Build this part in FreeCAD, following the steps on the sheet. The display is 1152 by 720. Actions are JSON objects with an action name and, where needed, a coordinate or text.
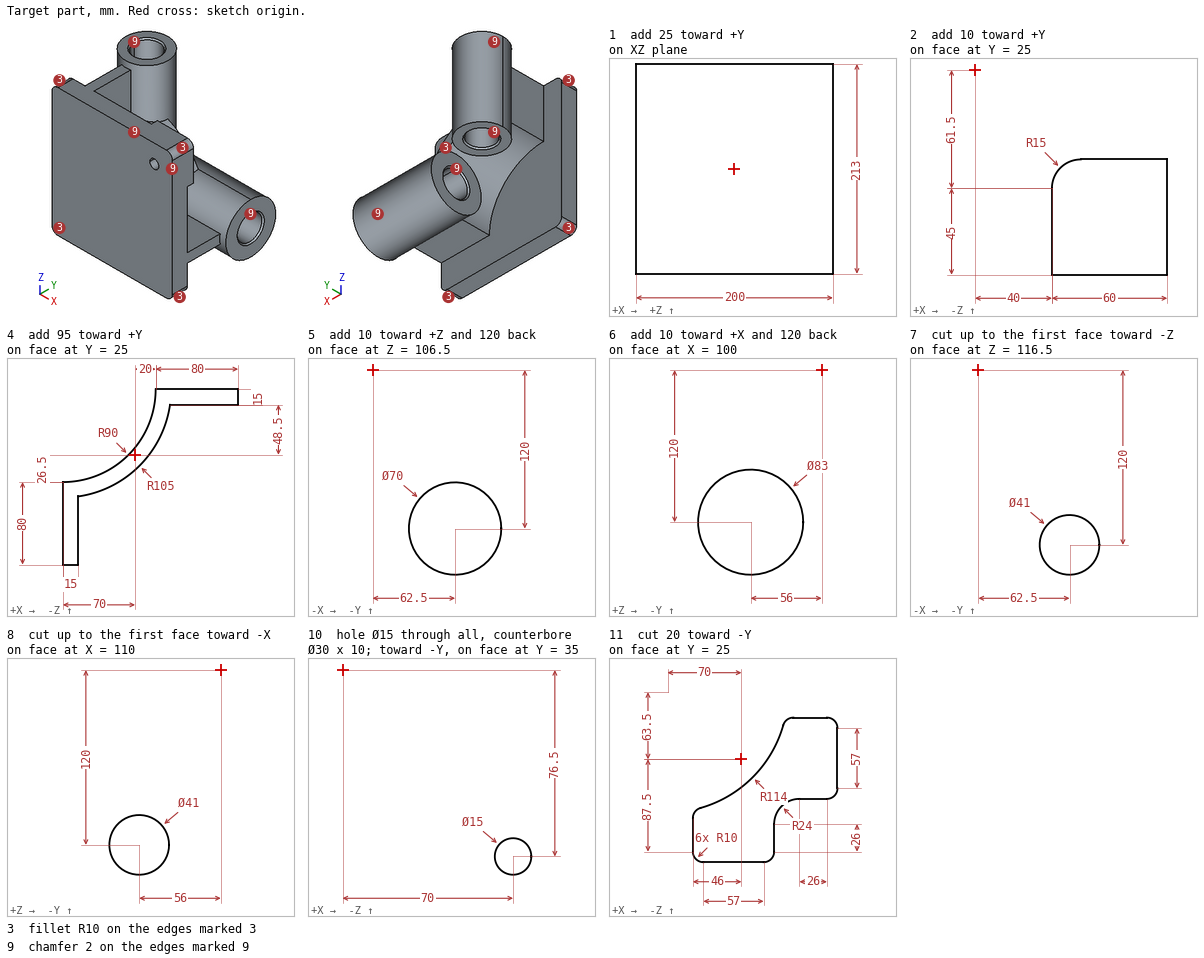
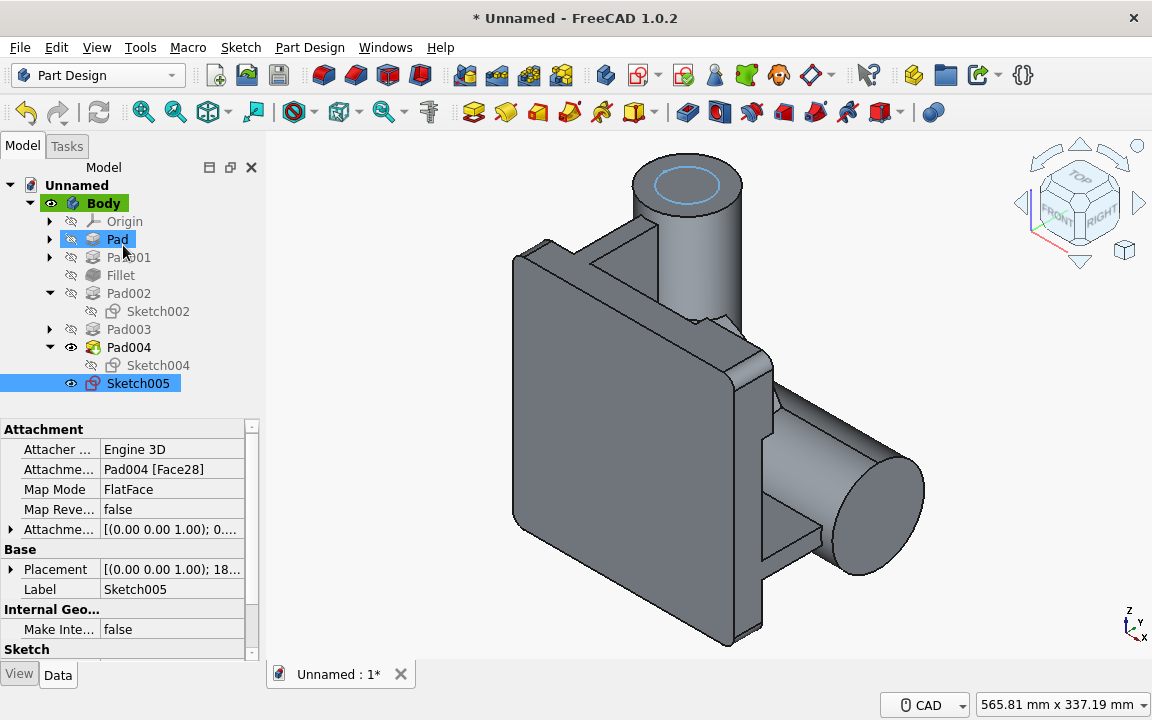
{"action": "left_click", "coordinate": [688, 112]}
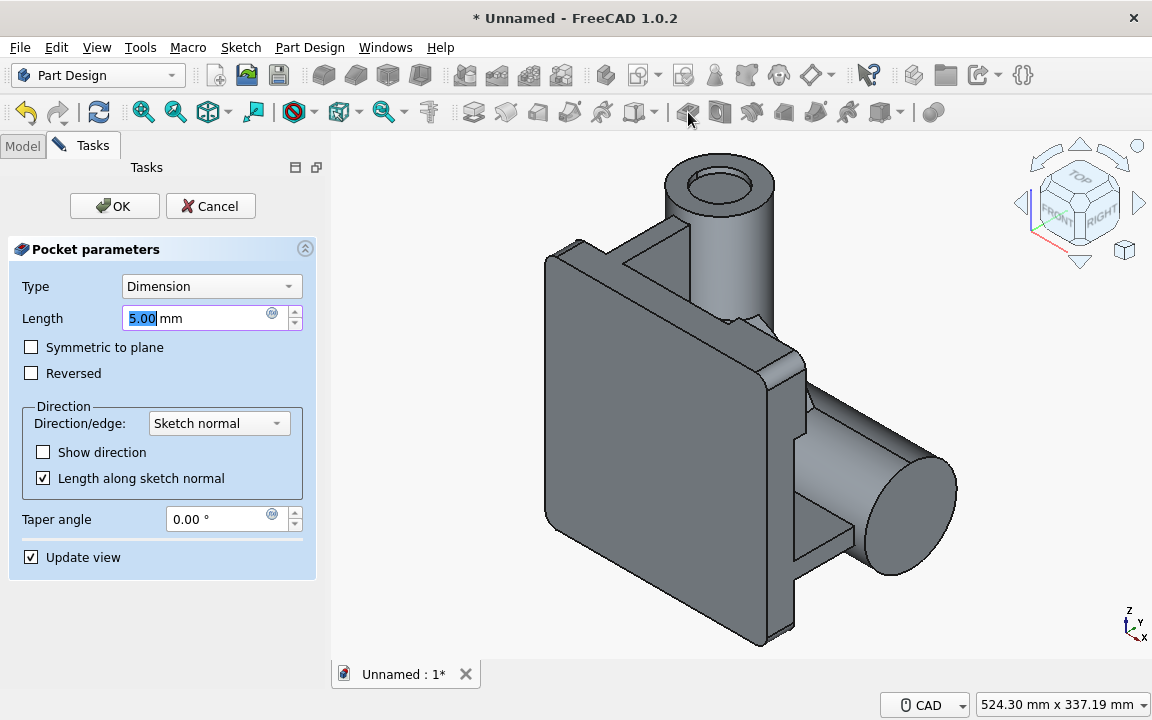
{"action": "left_click", "coordinate": [212, 286]}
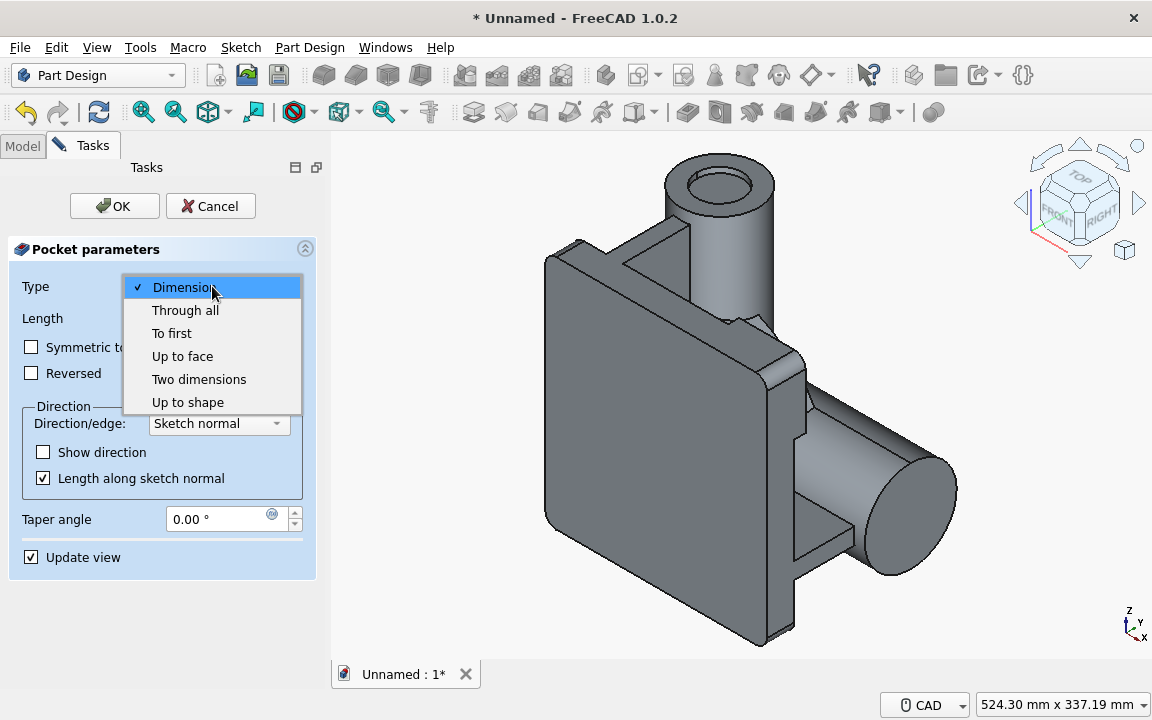
{"action": "left_click", "coordinate": [212, 334]}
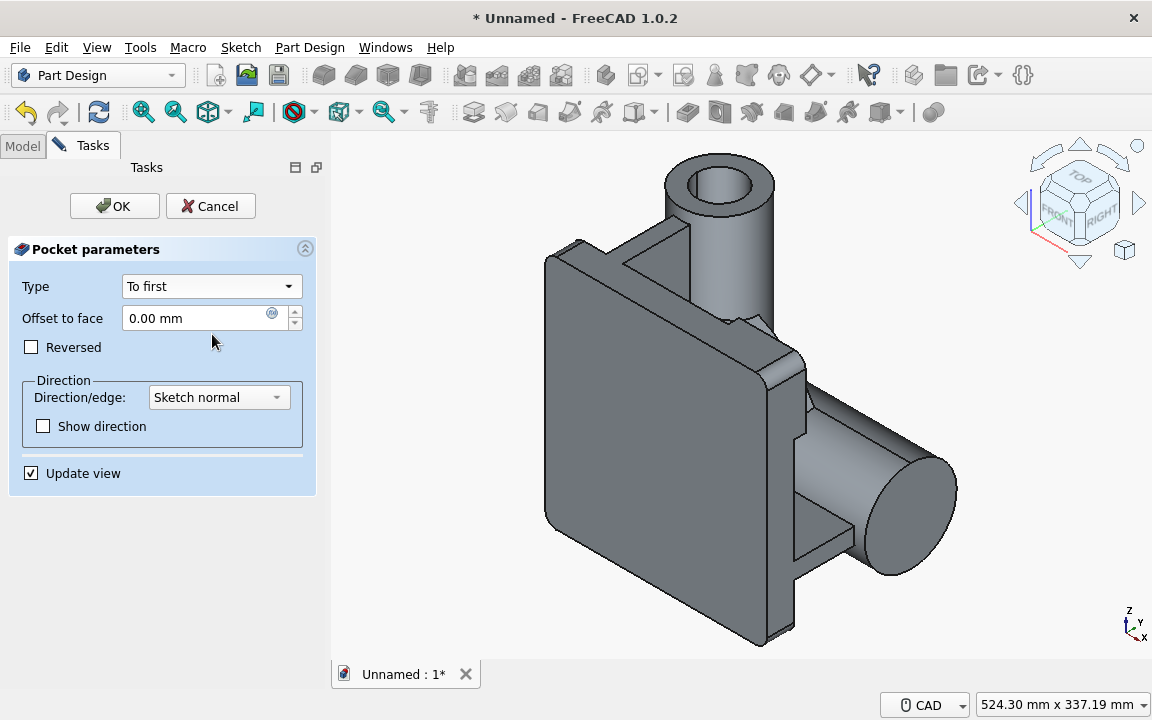
{"action": "left_click", "coordinate": [115, 206]}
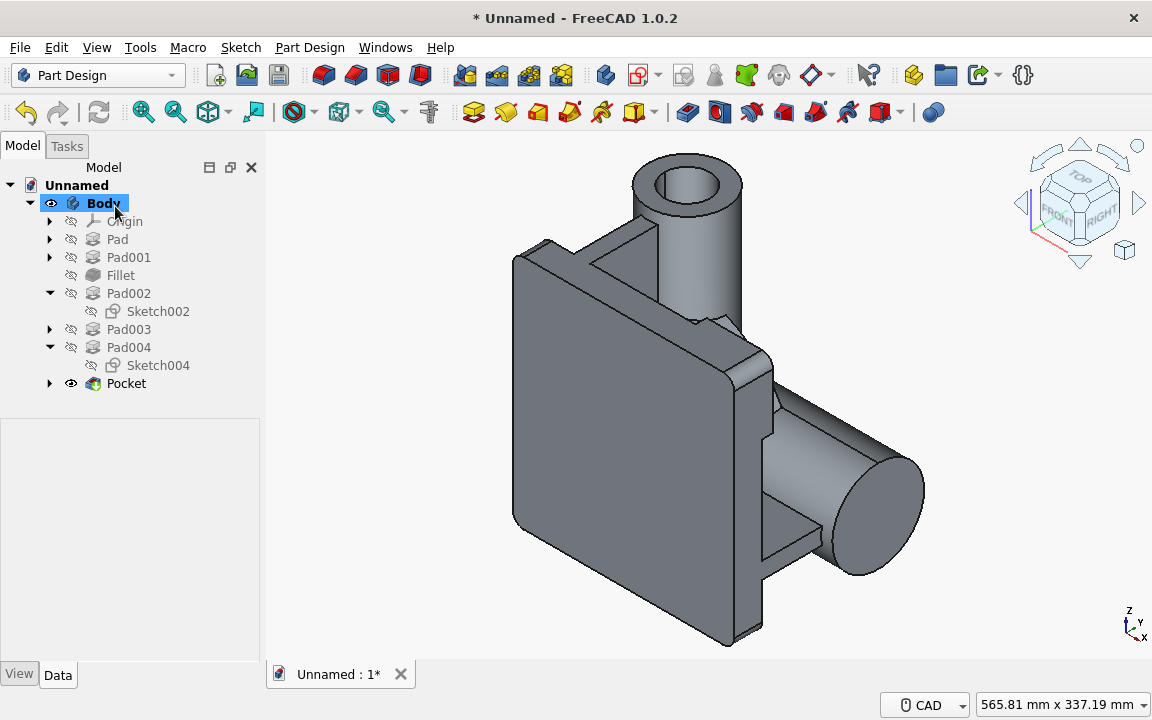
{"action": "left_click", "coordinate": [878, 515]}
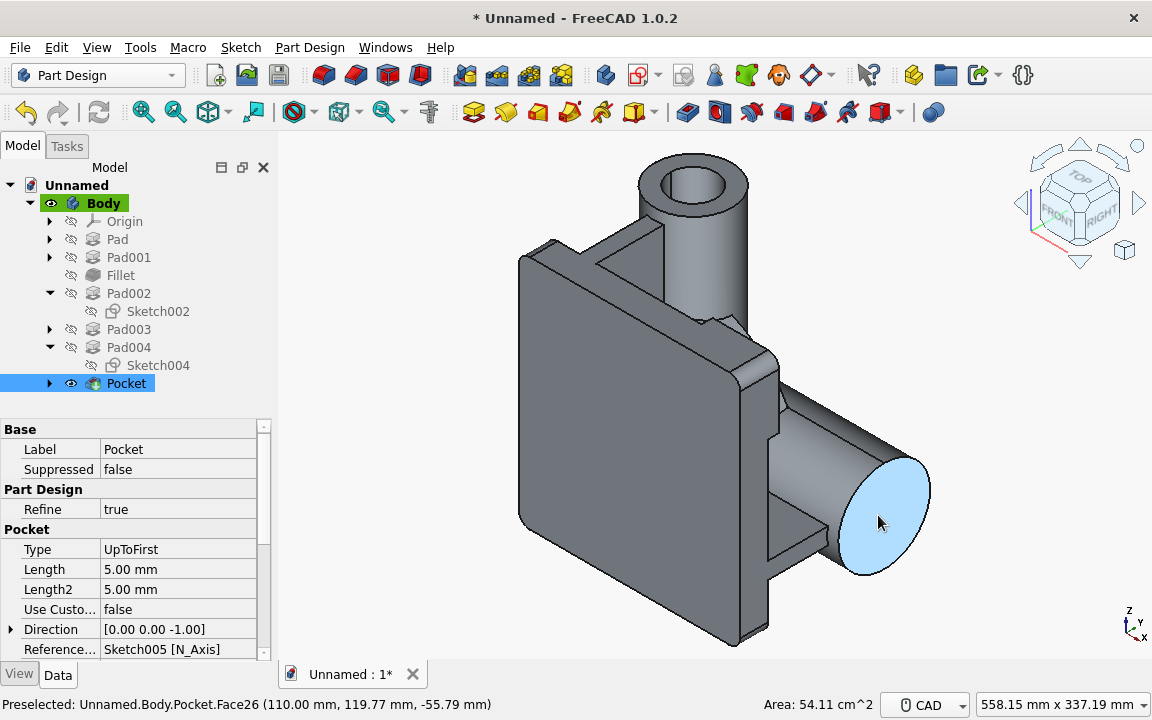
{"action": "left_click", "coordinate": [638, 76]}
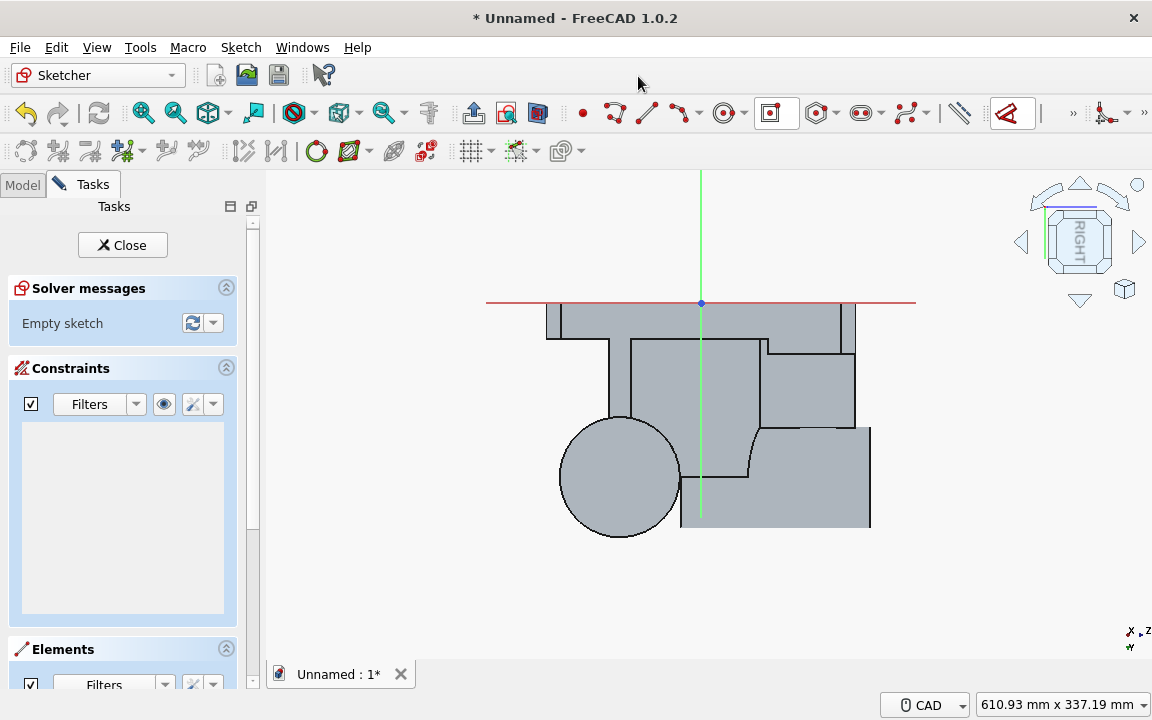
{"action": "scroll", "coordinate": [615, 493], "scroll_direction": "up", "scroll_amount": 8}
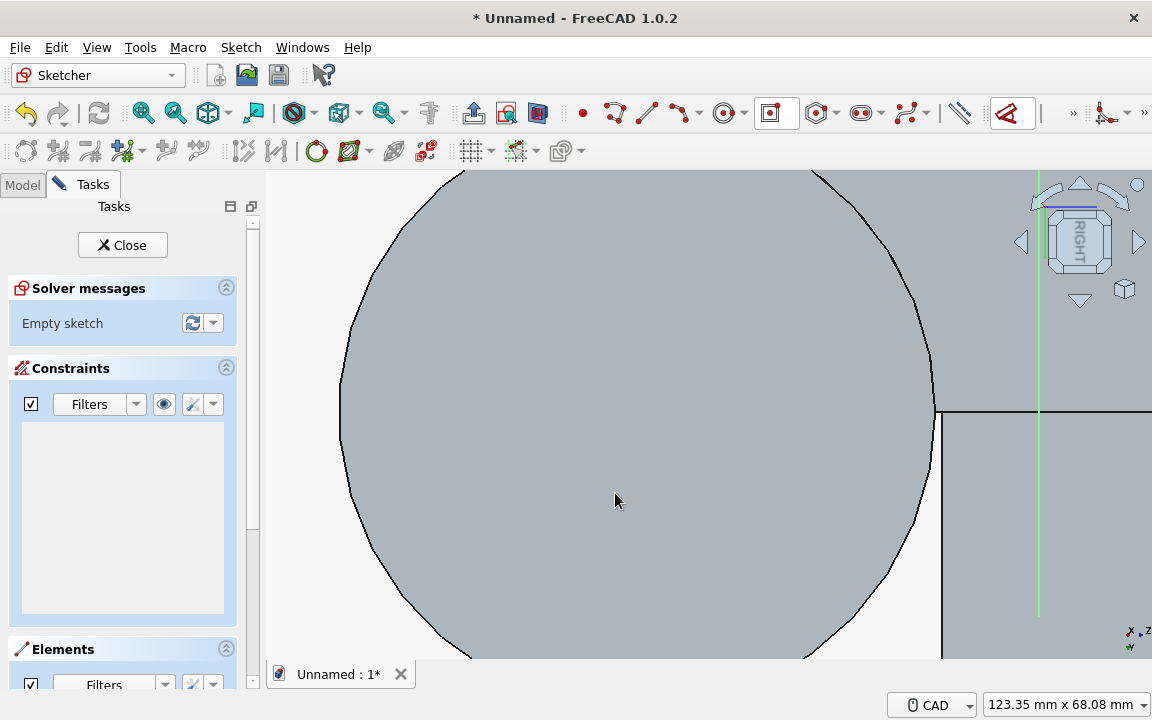
{"action": "left_click", "coordinate": [724, 114]}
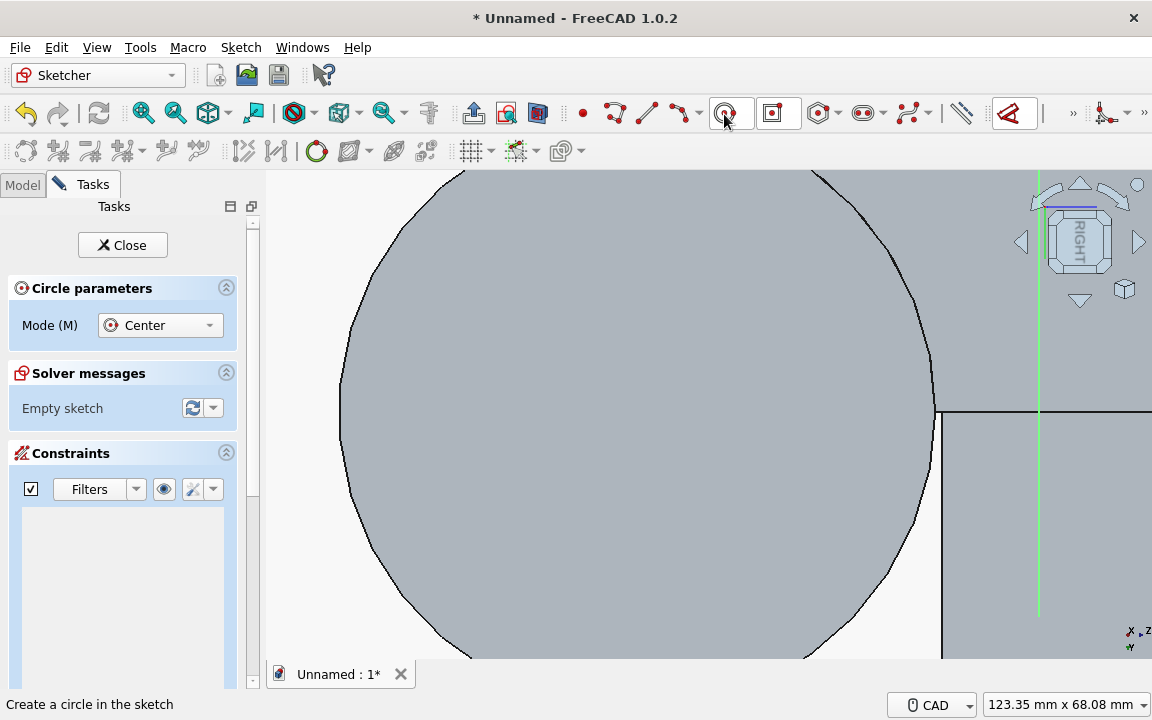
{"action": "left_click", "coordinate": [637, 412]}
{"action": "mouse_move", "coordinate": [741, 308]}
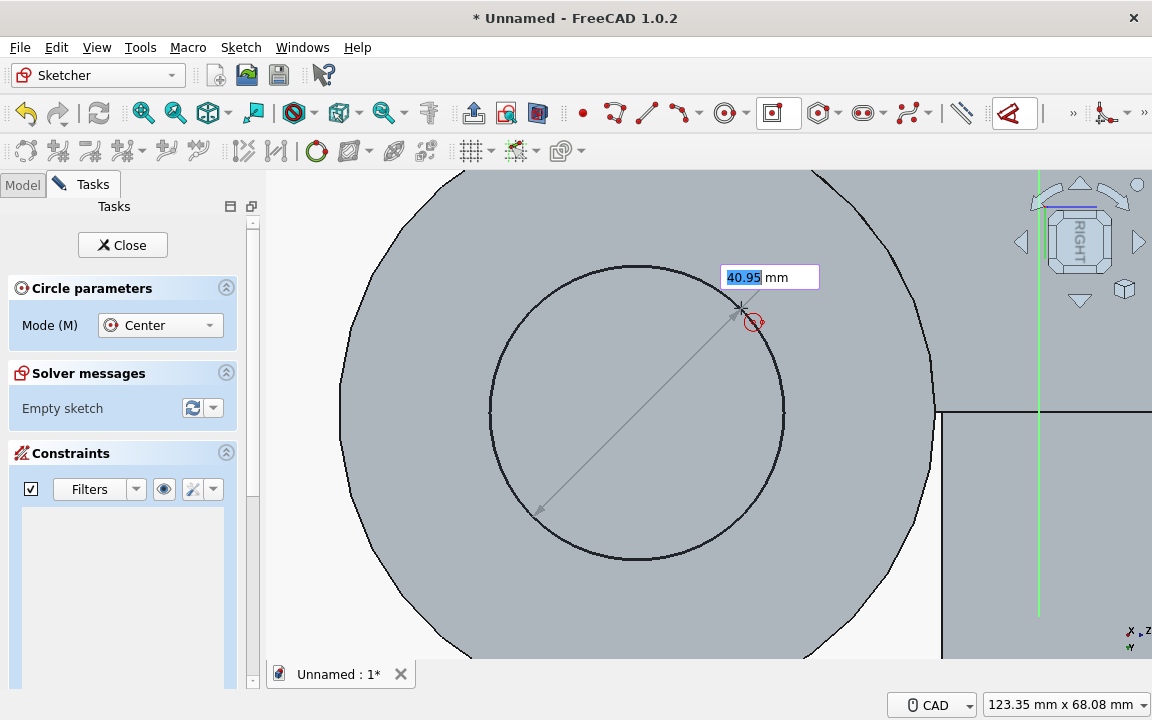
{"action": "type", "text": "41"}
{"action": "key", "text": "Return"}
{"action": "key", "text": "Escape"}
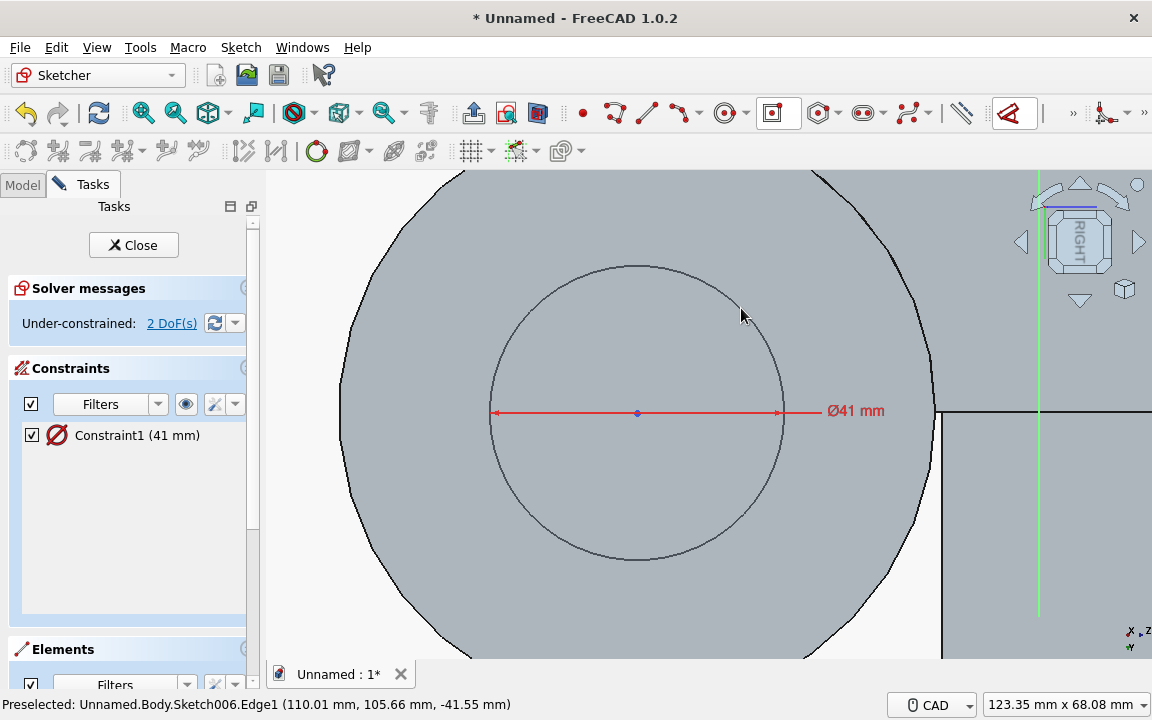
{"action": "left_click", "coordinate": [637, 413]}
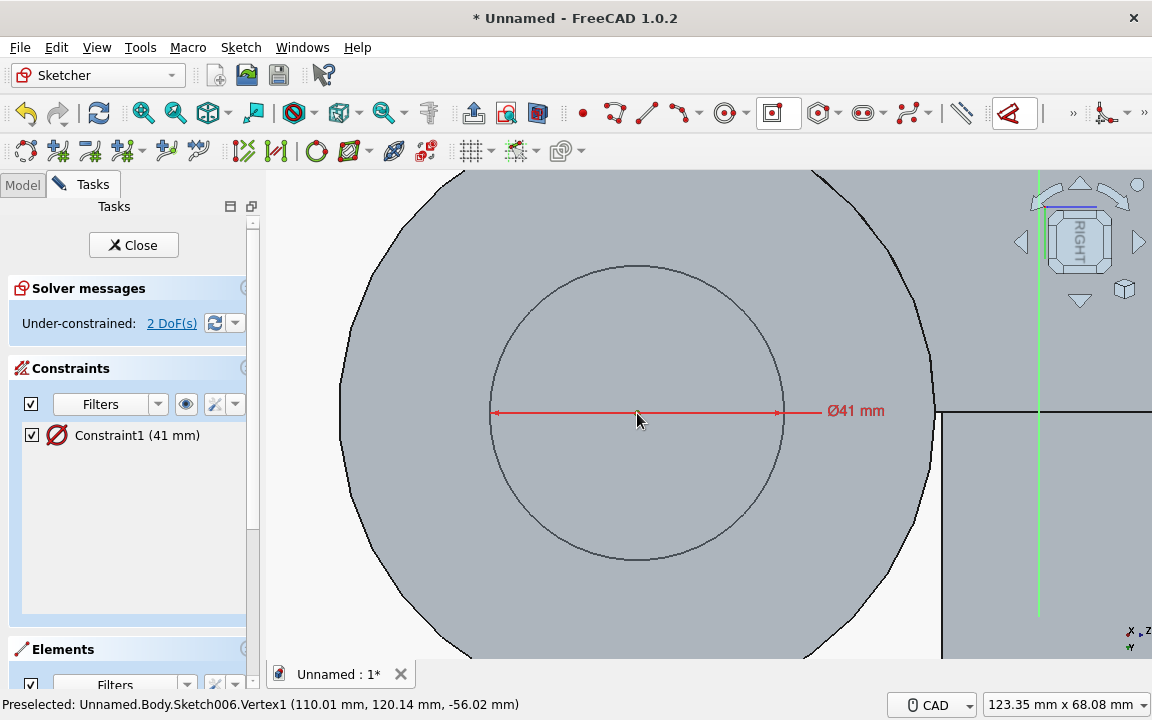
{"action": "key", "text": "l"}